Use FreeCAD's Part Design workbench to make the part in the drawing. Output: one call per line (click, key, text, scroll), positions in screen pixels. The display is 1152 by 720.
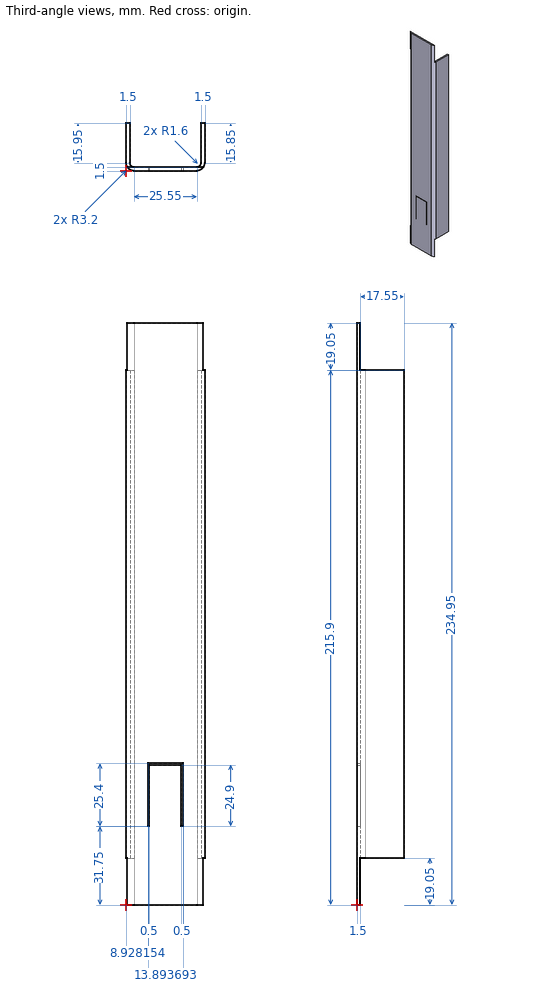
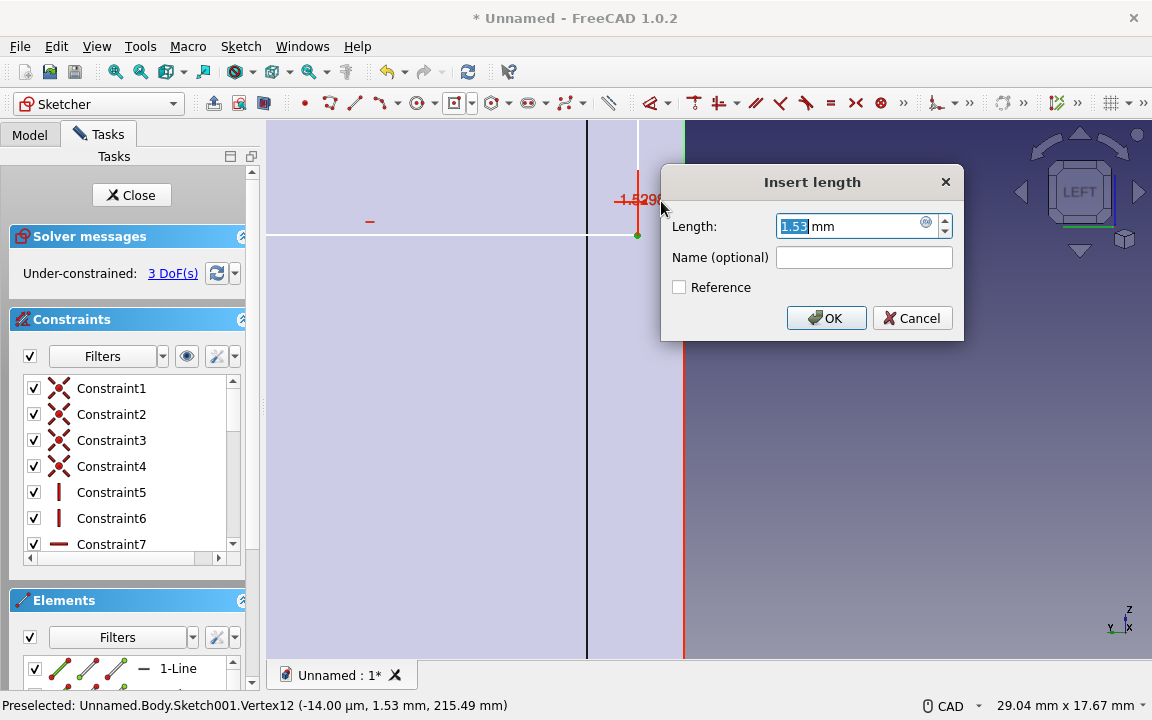
text(1.5)
key(Return)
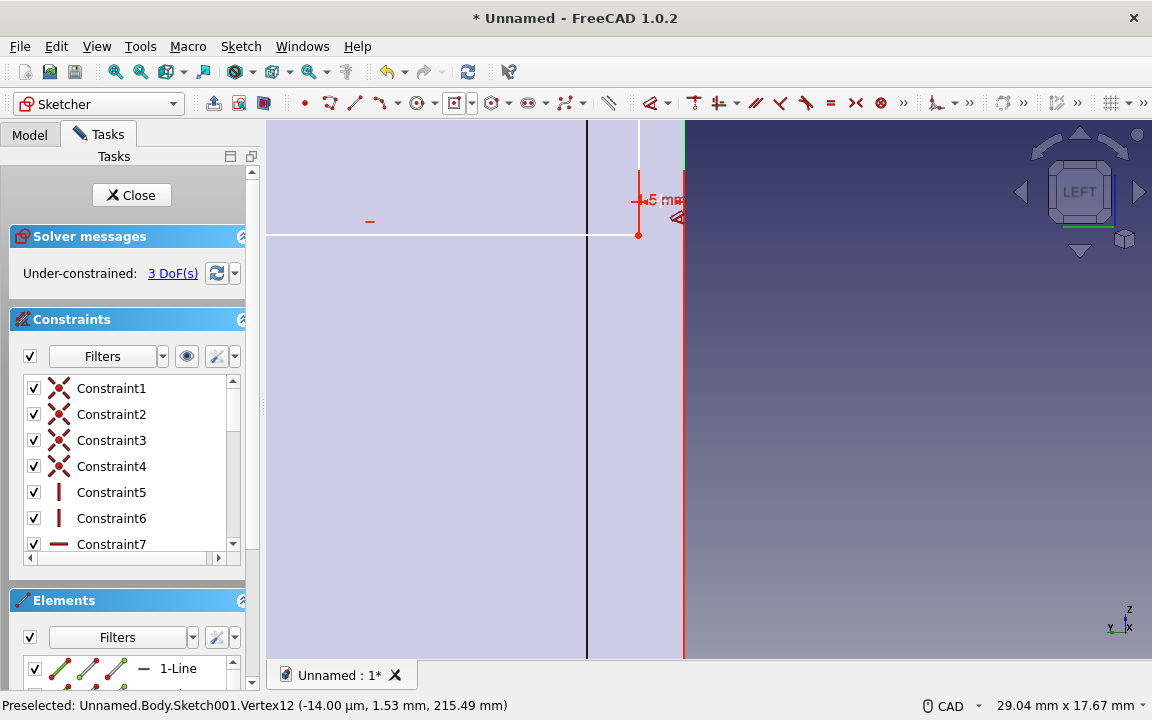
scroll(653, 241, down, 15)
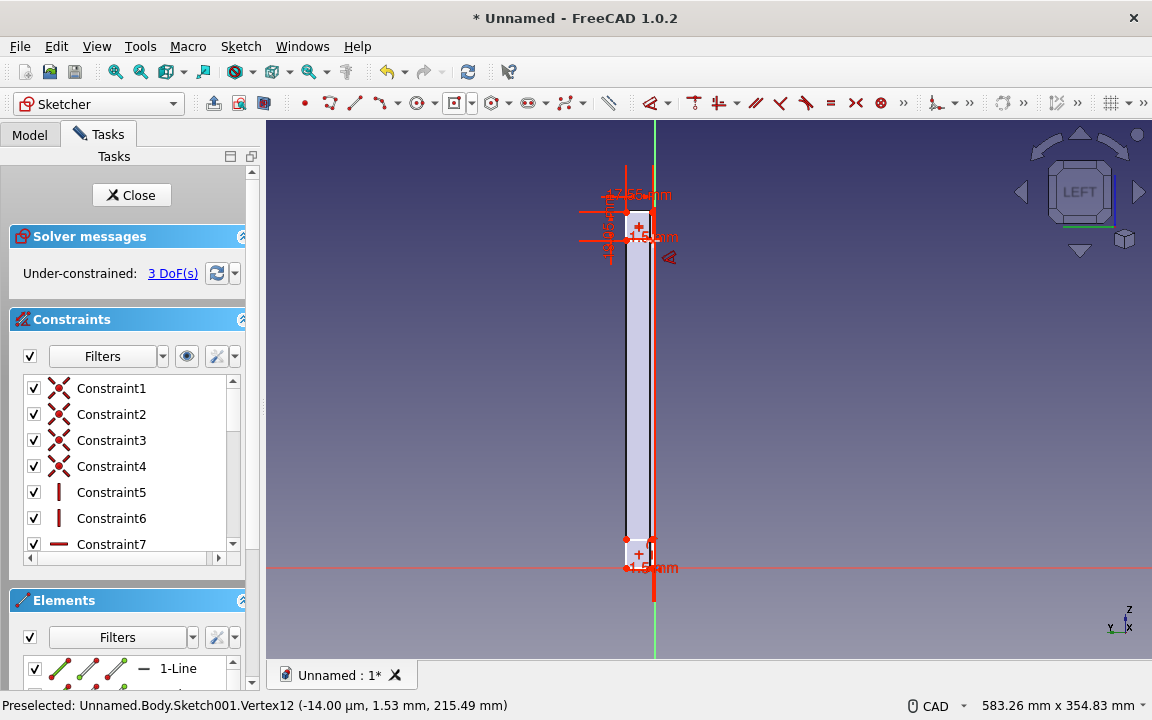
scroll(626, 548, up, 3)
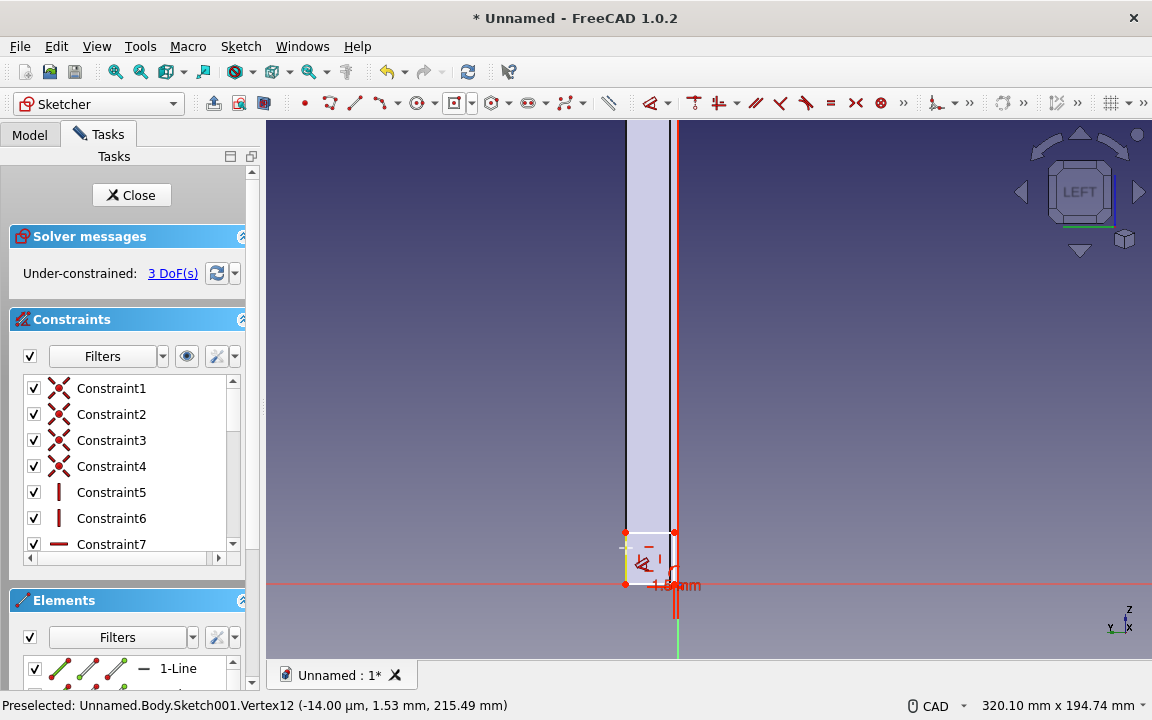
click(626, 548)
click(592, 559)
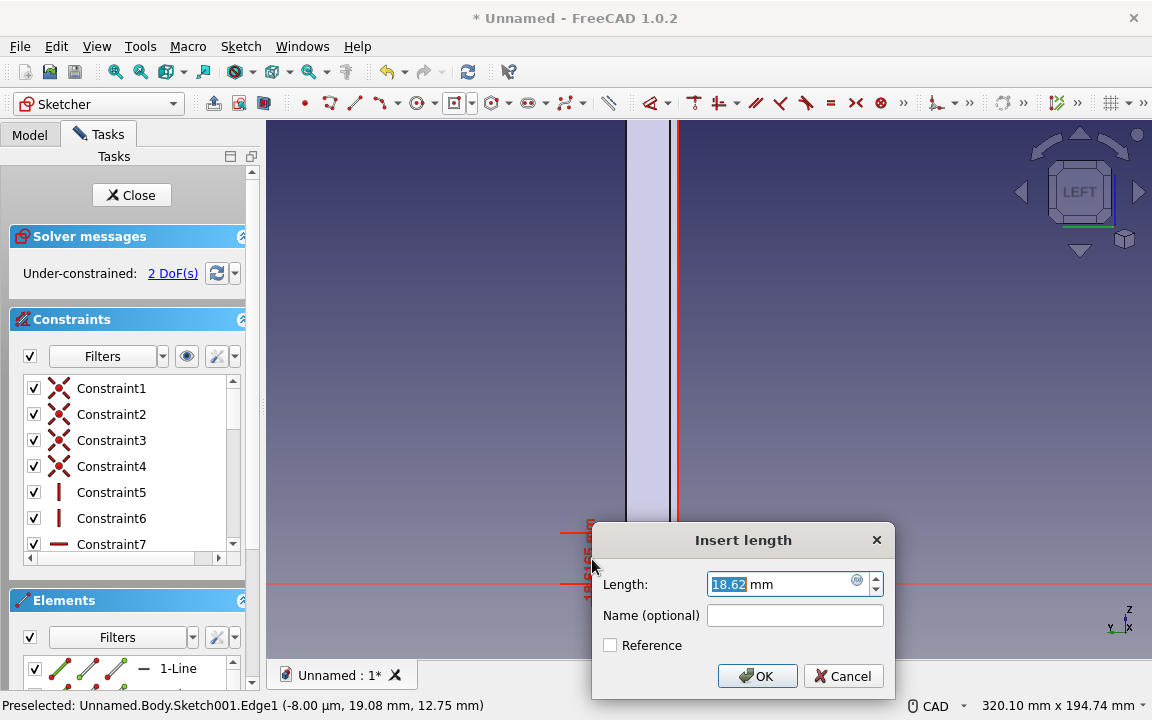
text(19.05)
key(Return)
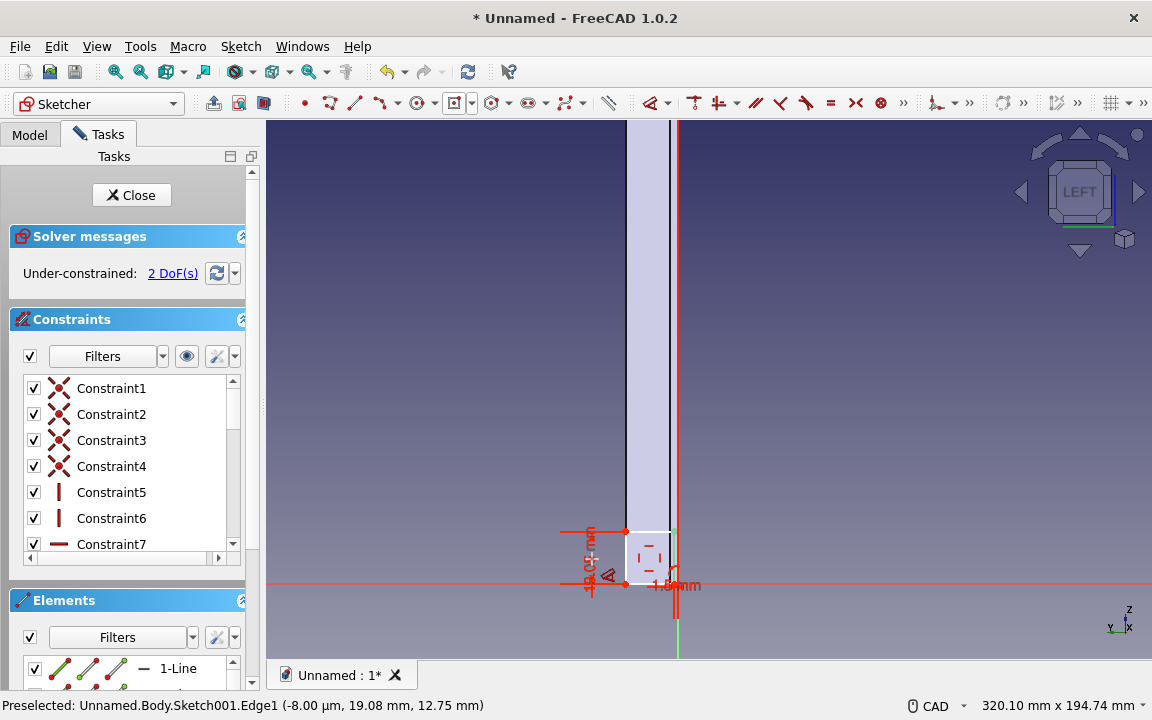
click(640, 584)
click(650, 618)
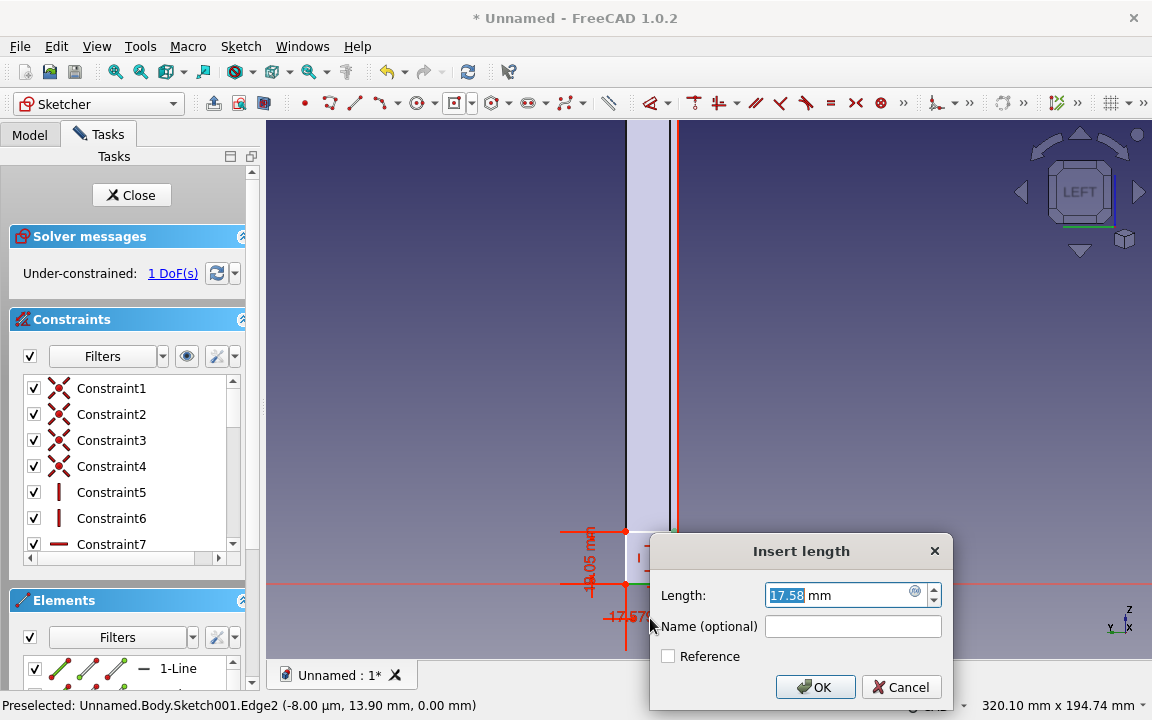
text(17.55)
key(Return)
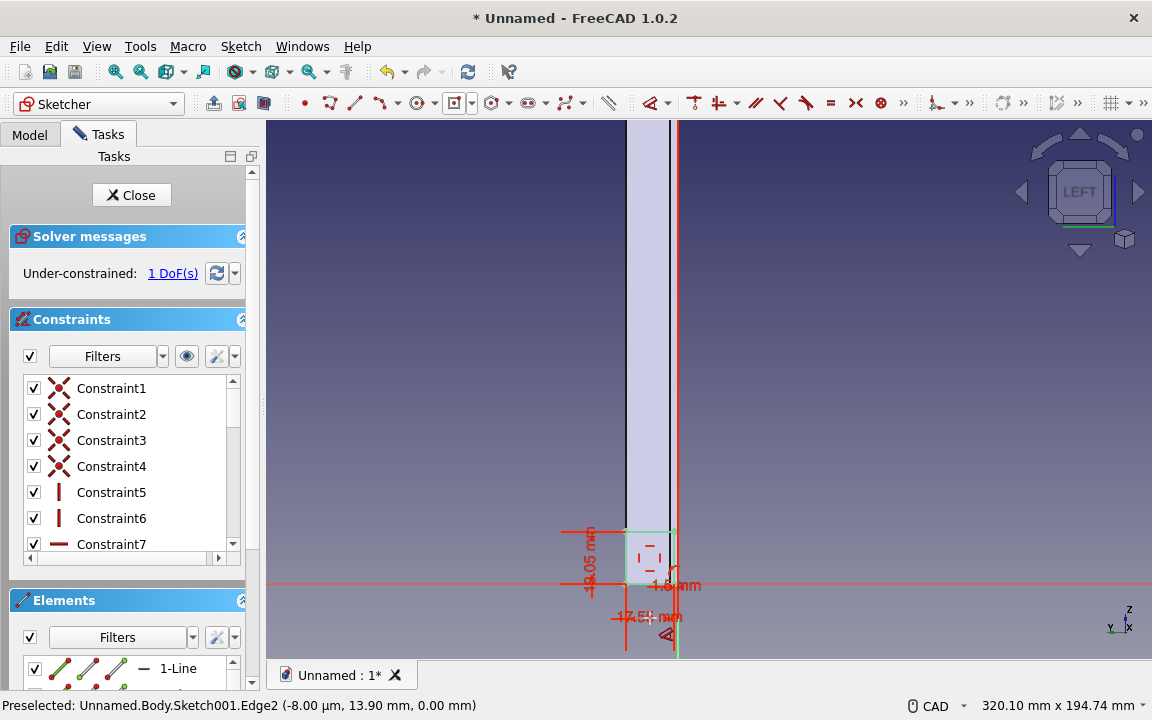
scroll(626, 548, down, 3)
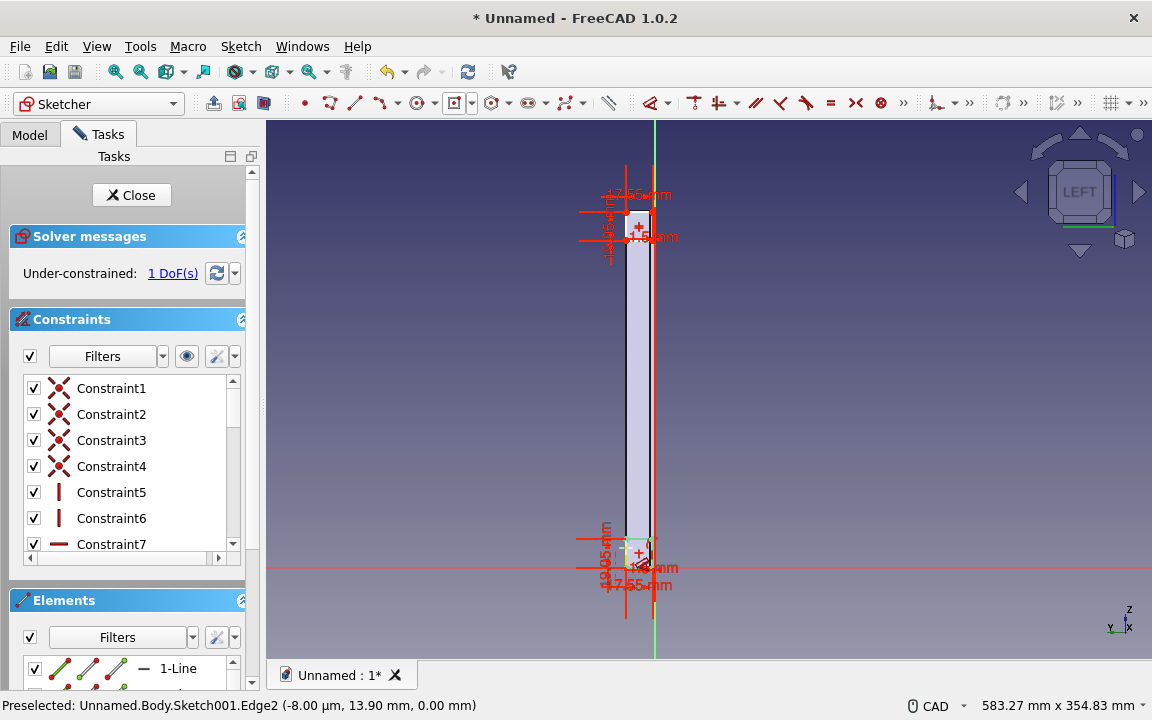
click(626, 241)
click(592, 405)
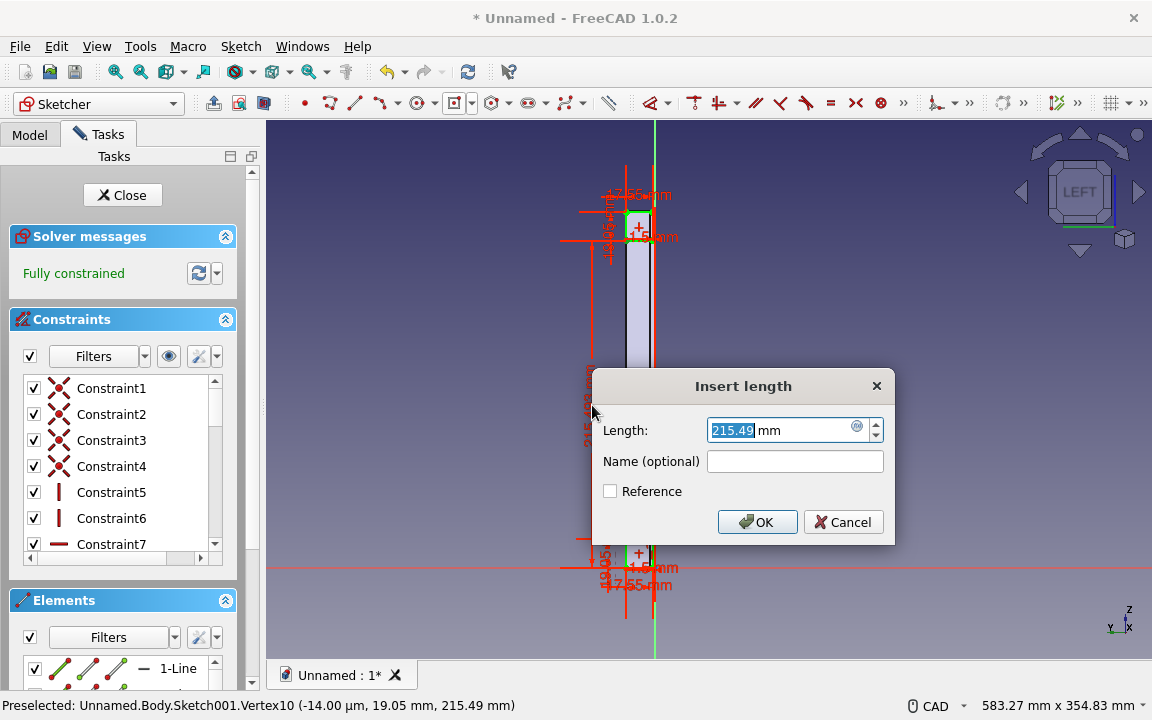
text(215.9)
key(Return)
key(Escape)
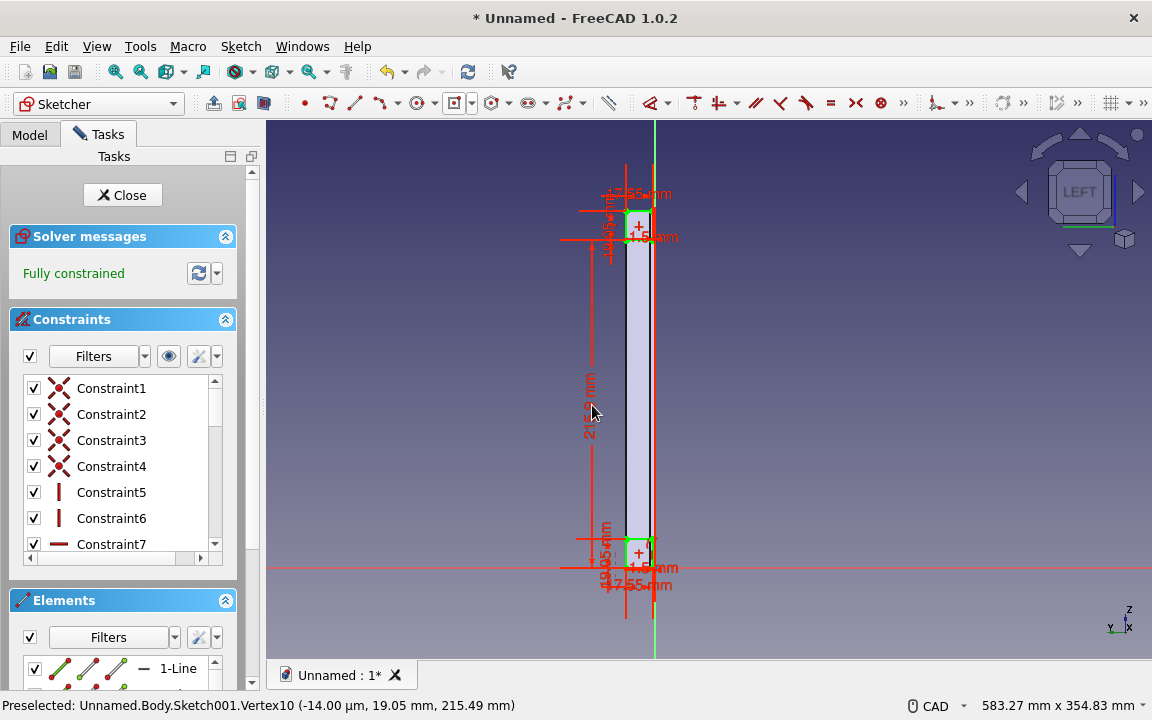
click(123, 195)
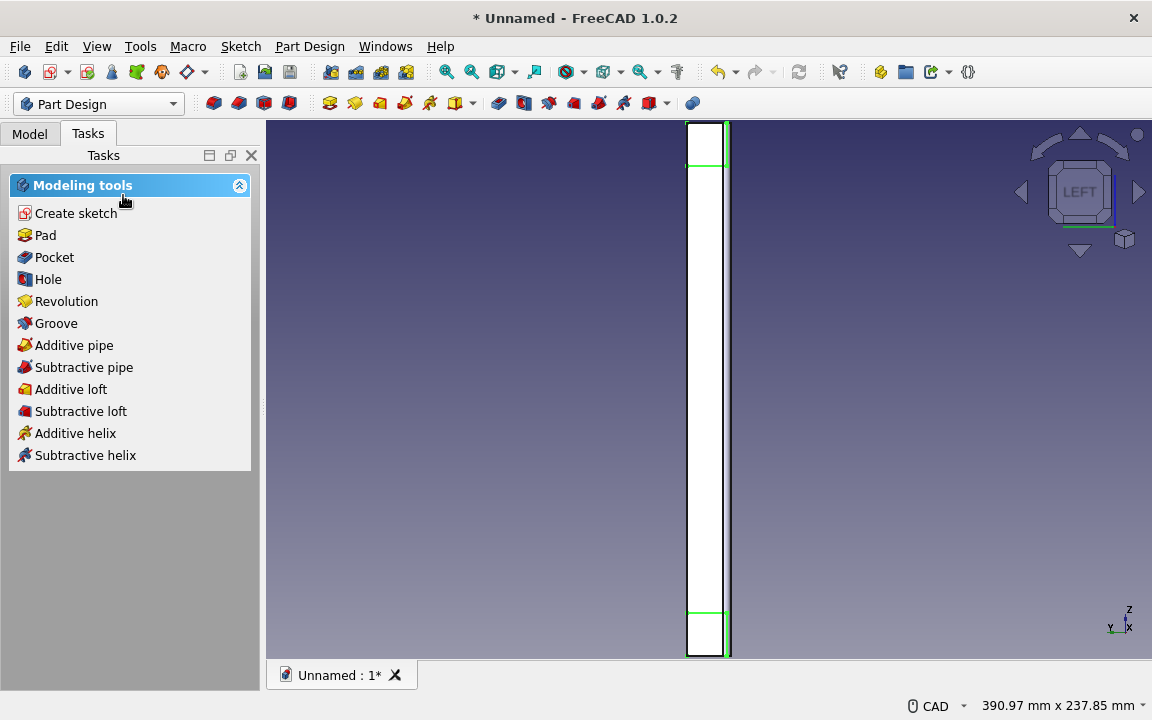
click(499, 104)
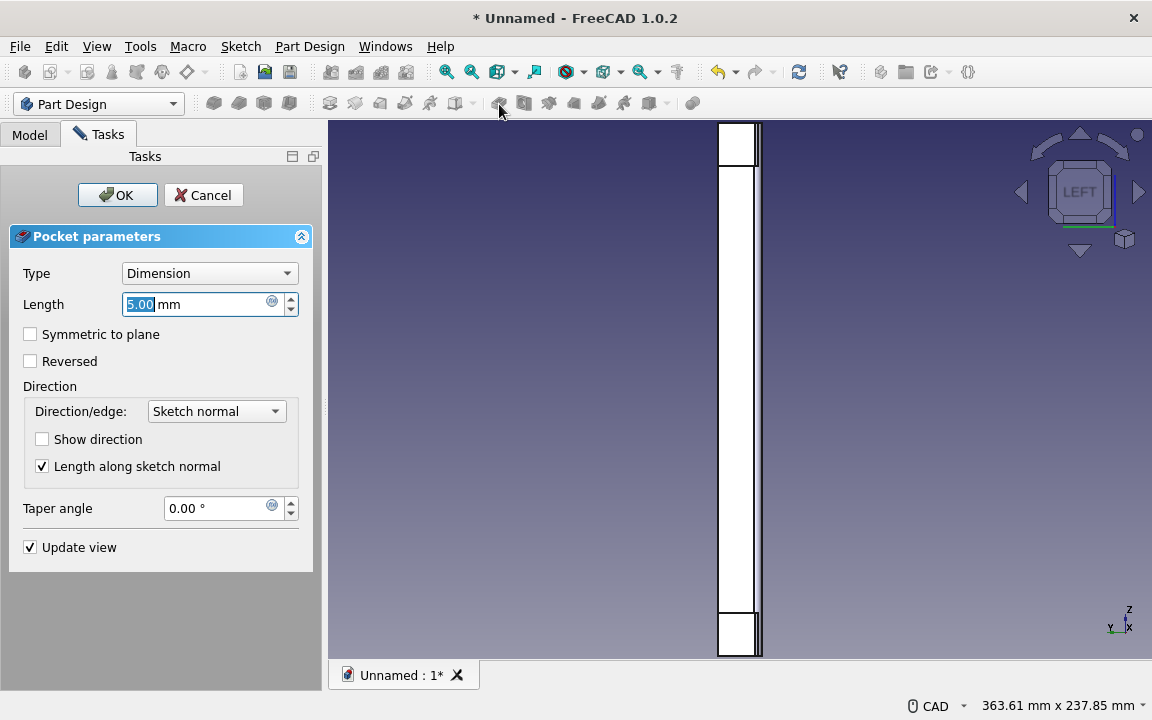
click(210, 274)